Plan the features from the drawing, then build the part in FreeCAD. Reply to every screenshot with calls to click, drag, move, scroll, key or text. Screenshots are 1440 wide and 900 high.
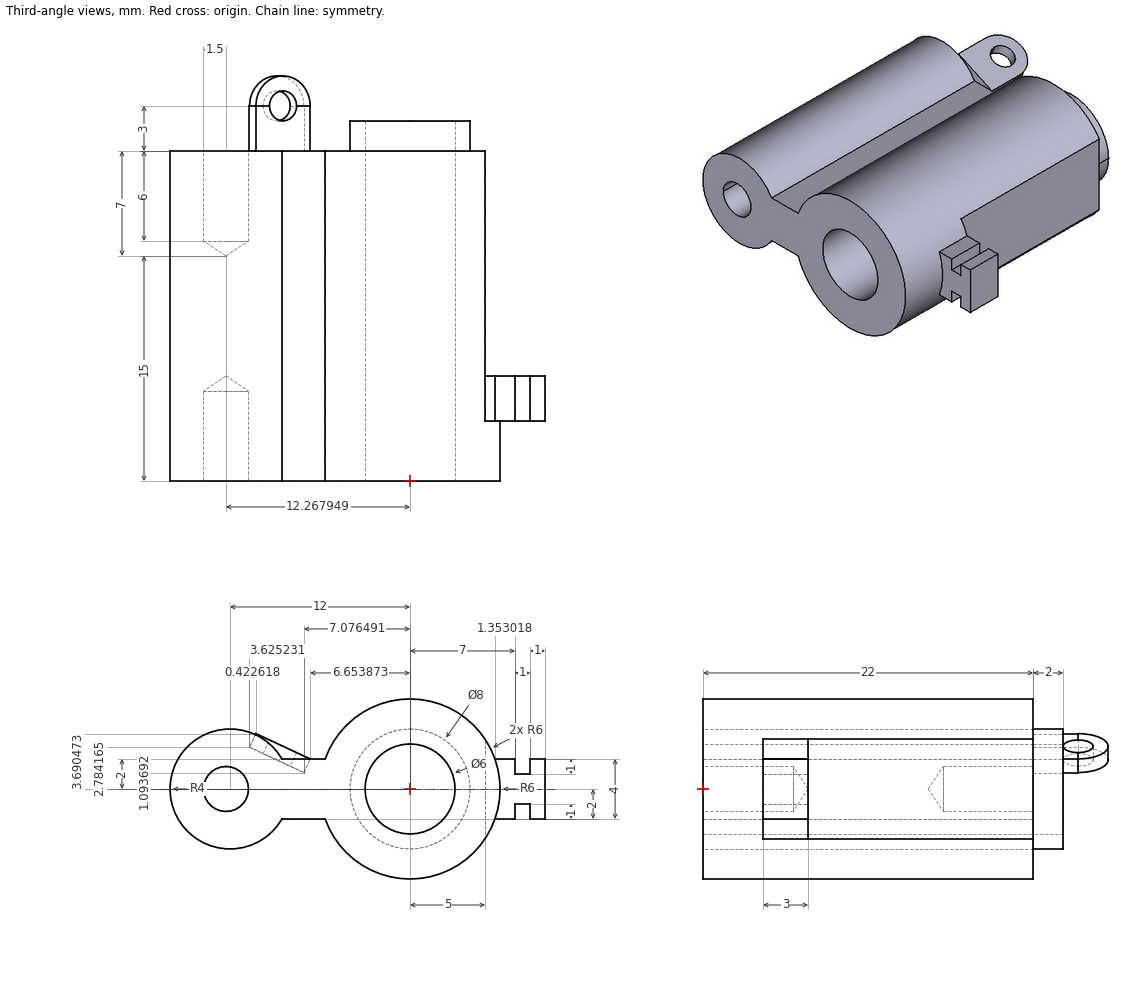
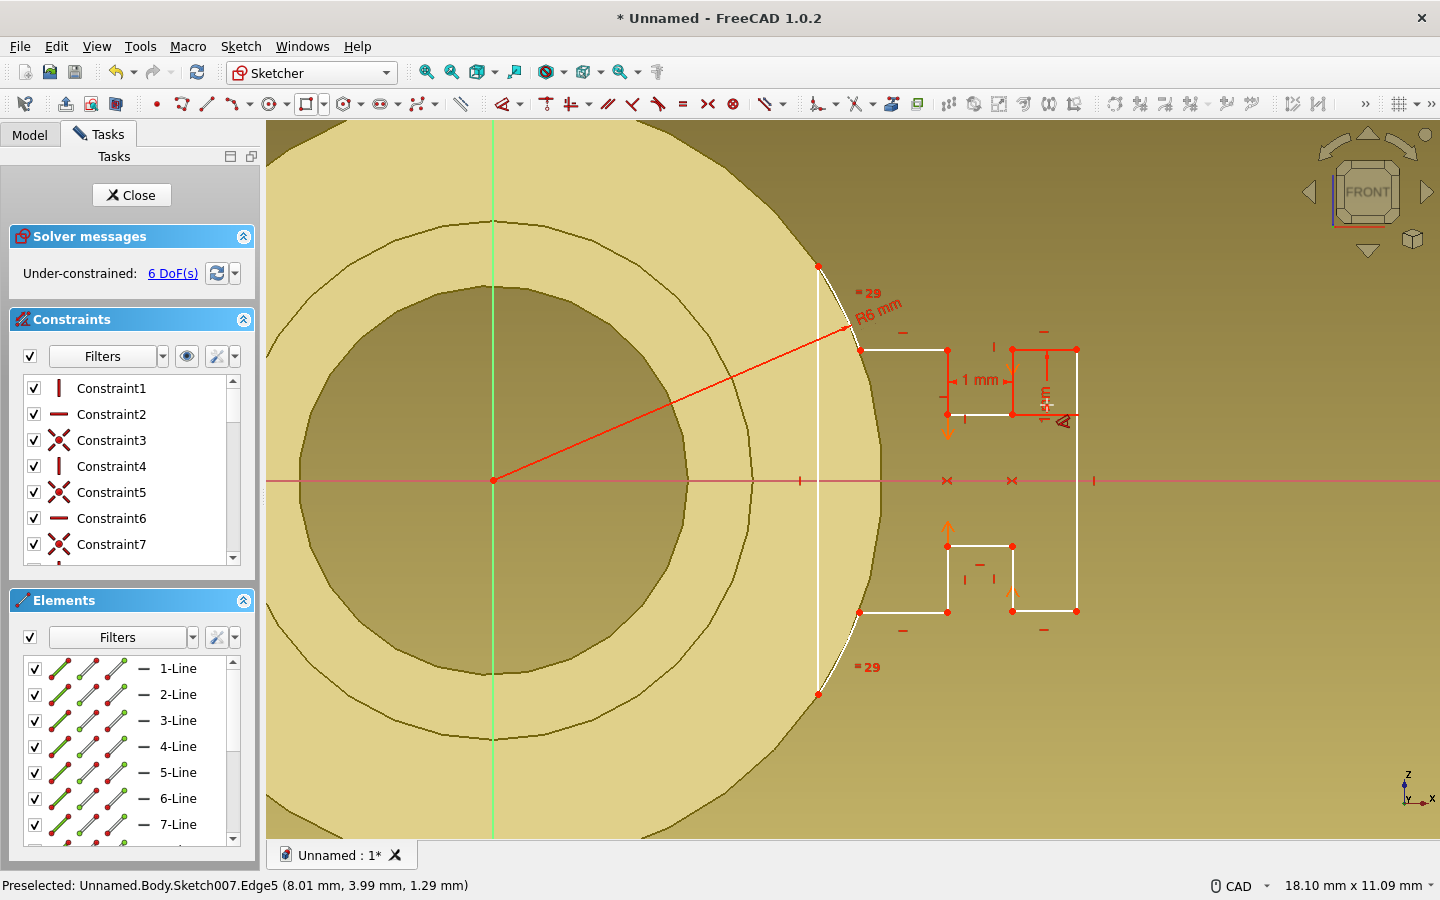
click(1032, 350)
click(1045, 316)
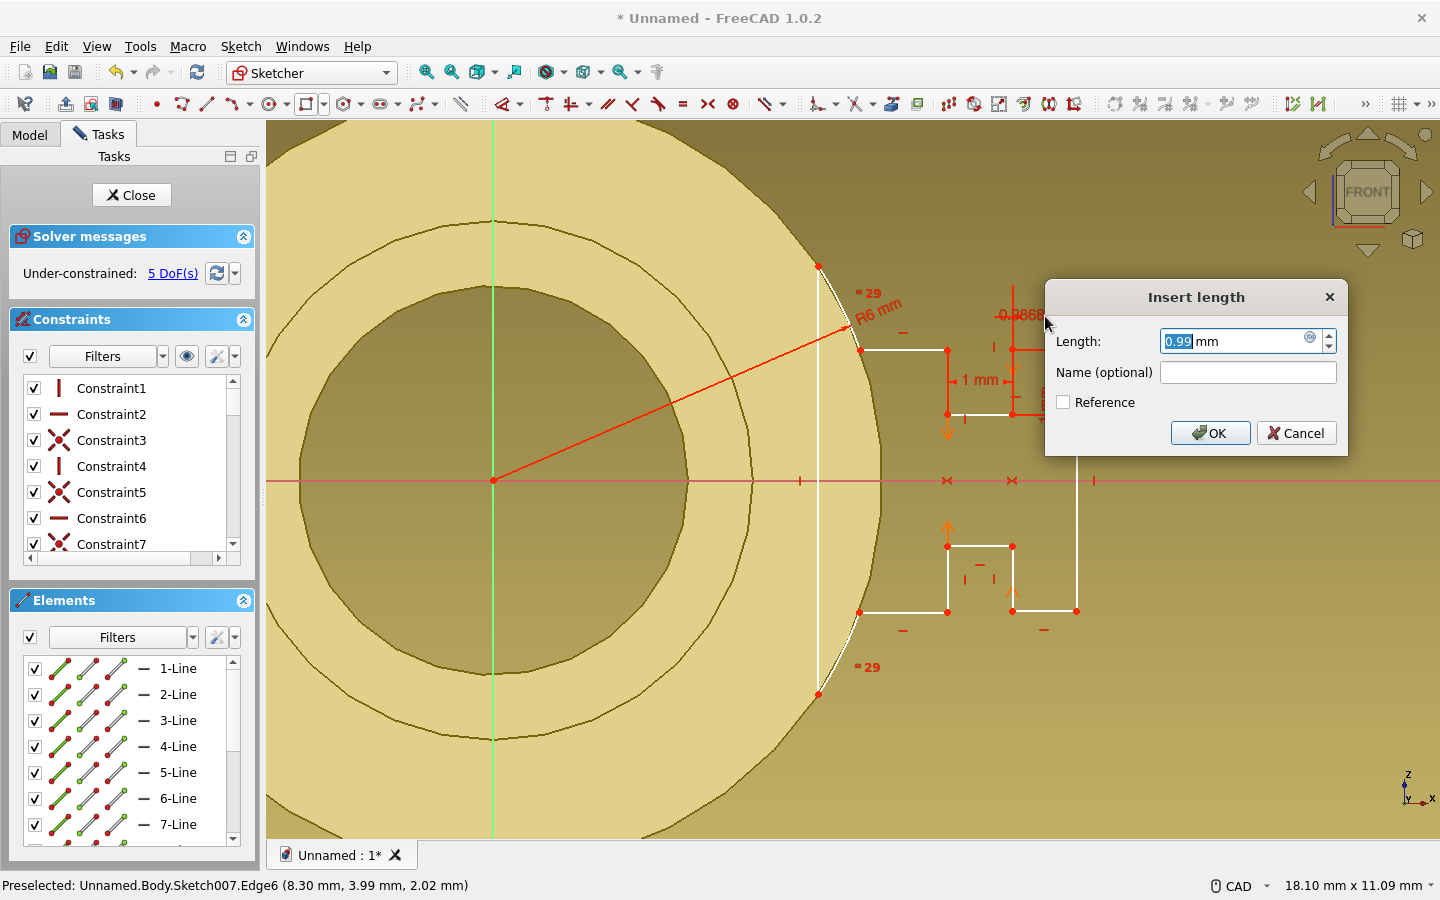
text(1)
key(Return)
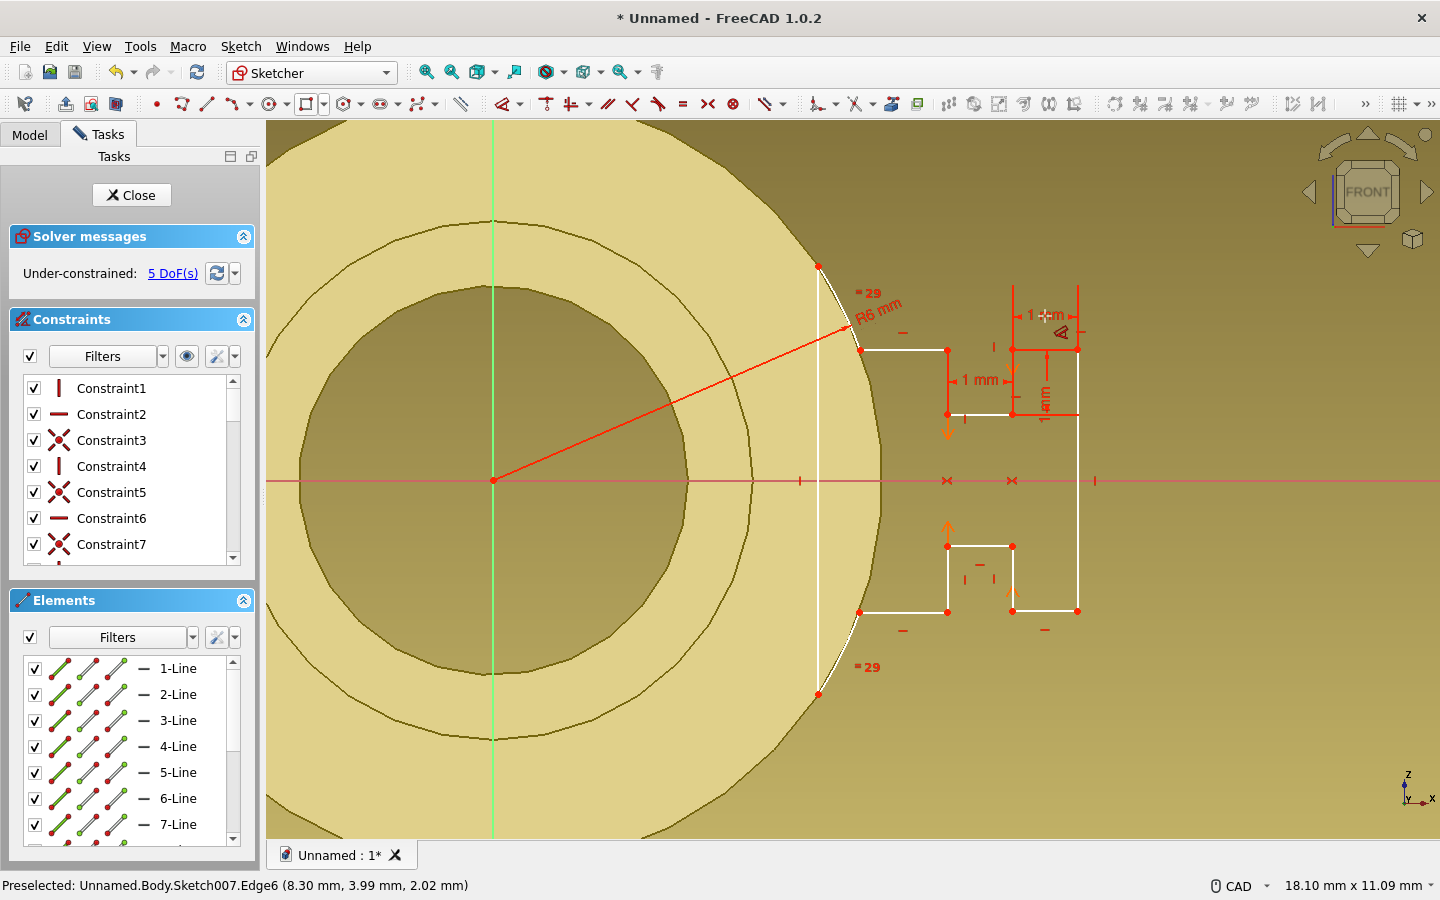
click(1078, 428)
click(1112, 541)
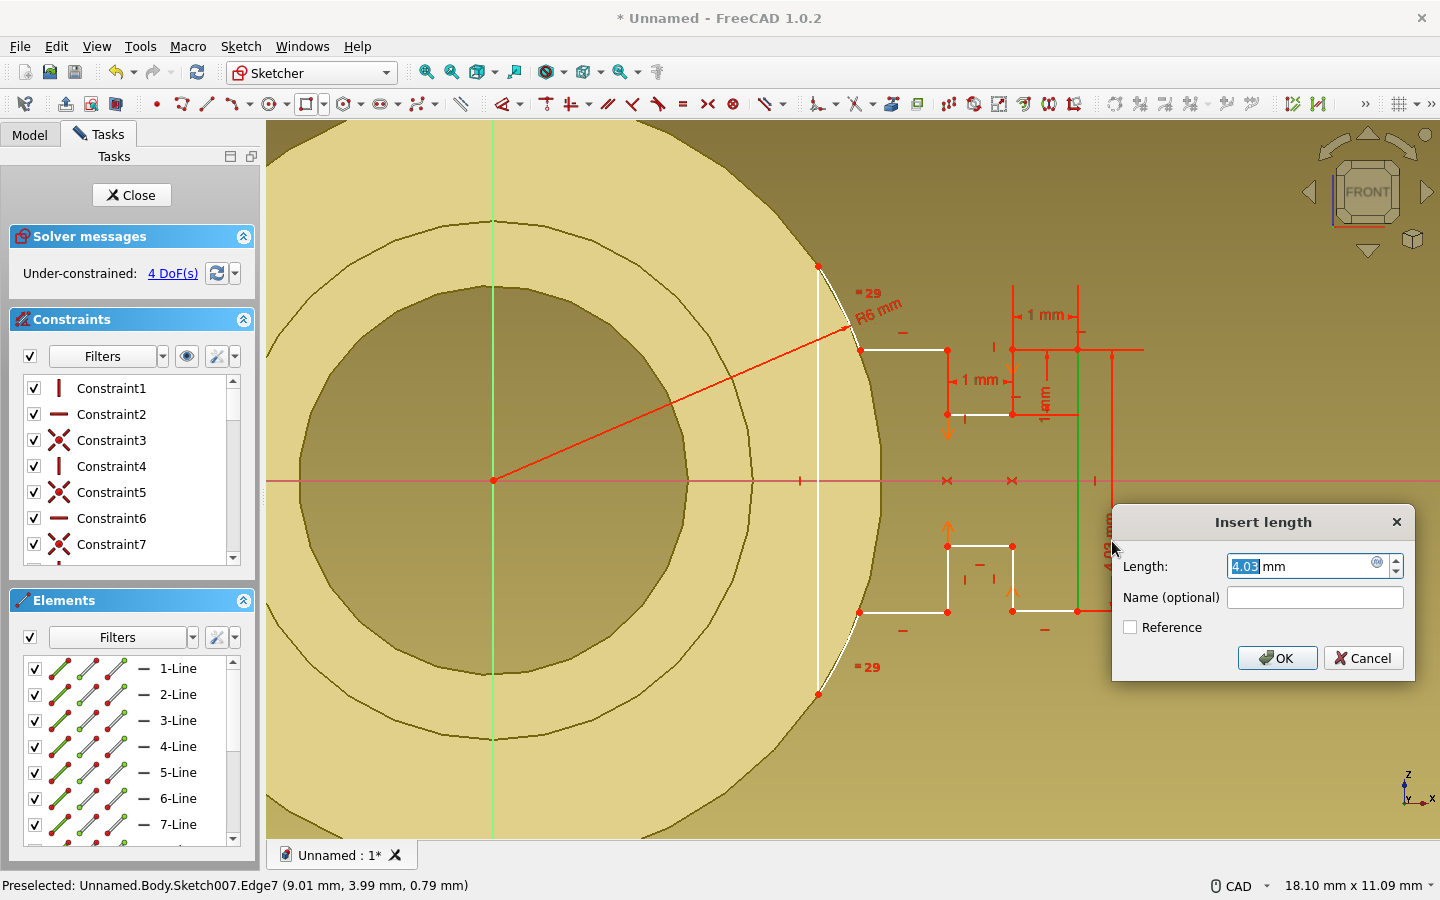
text(4)
key(Return)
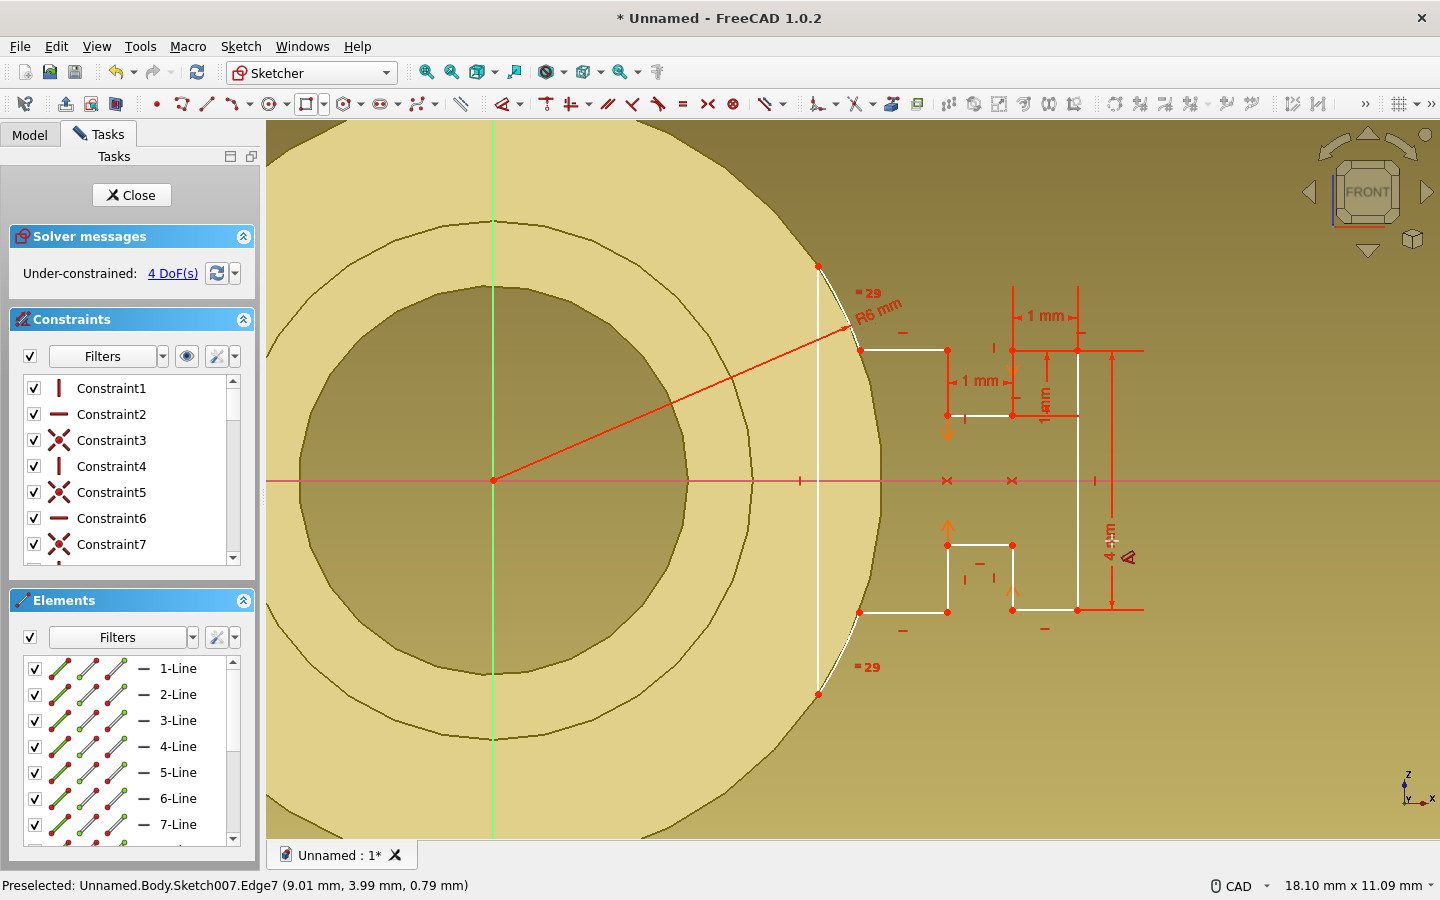
click(948, 566)
click(982, 579)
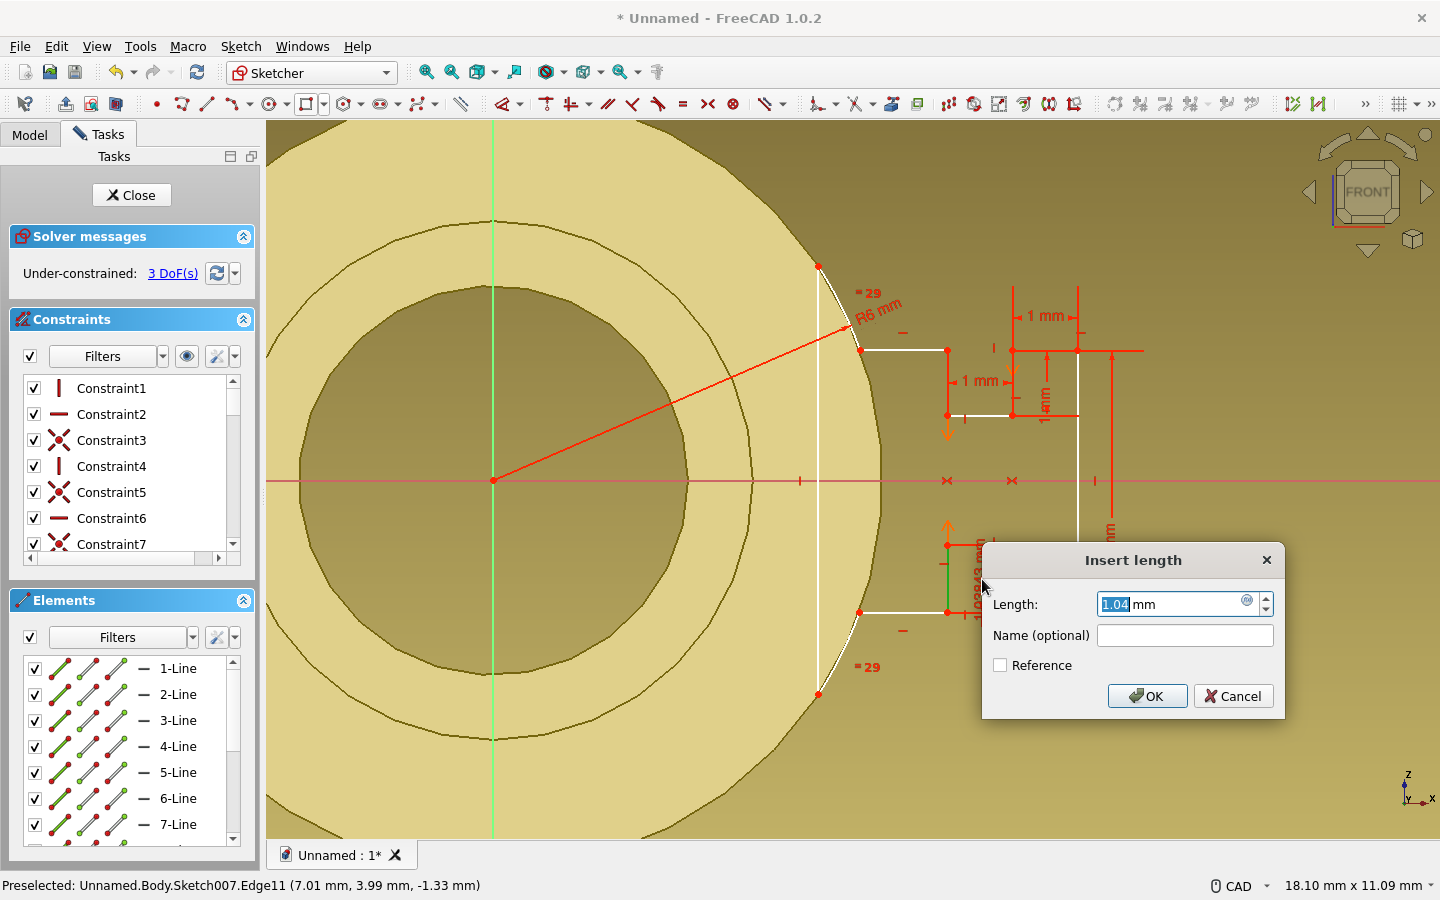
text(1)
key(Return)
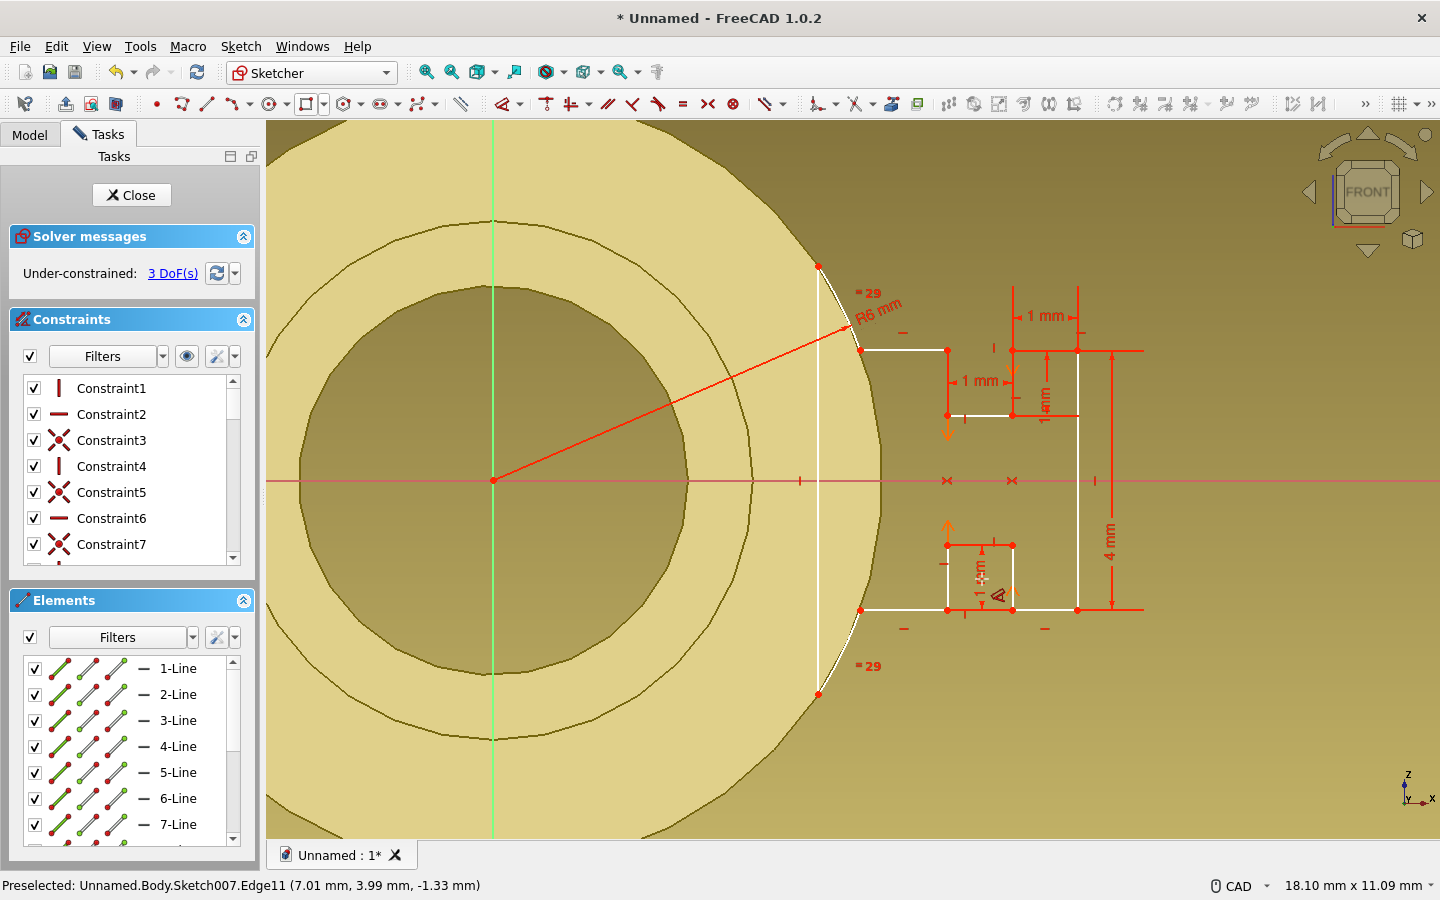
click(818, 695)
click(656, 729)